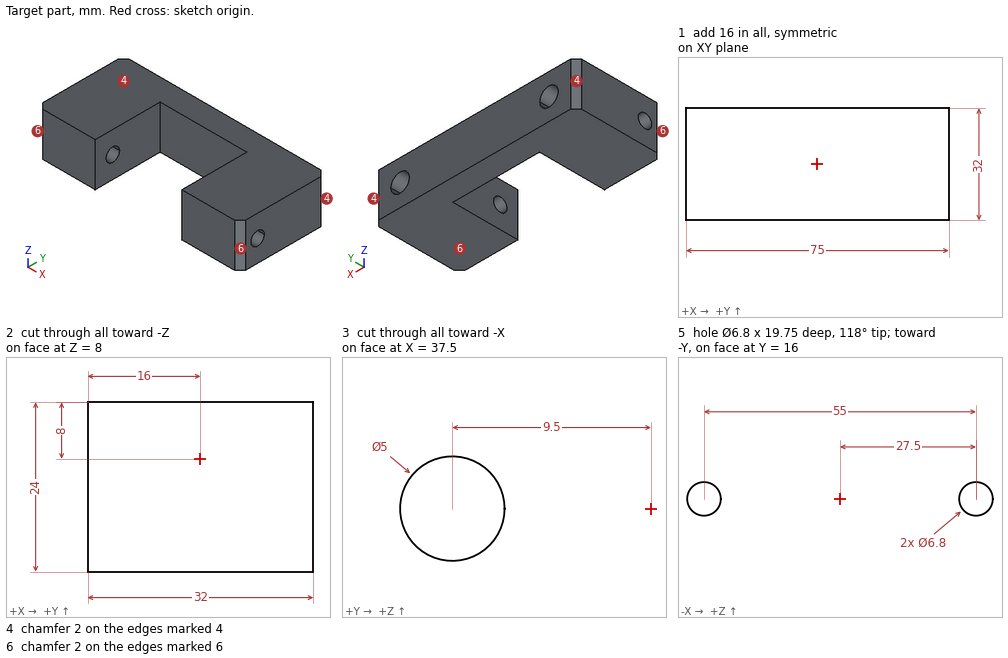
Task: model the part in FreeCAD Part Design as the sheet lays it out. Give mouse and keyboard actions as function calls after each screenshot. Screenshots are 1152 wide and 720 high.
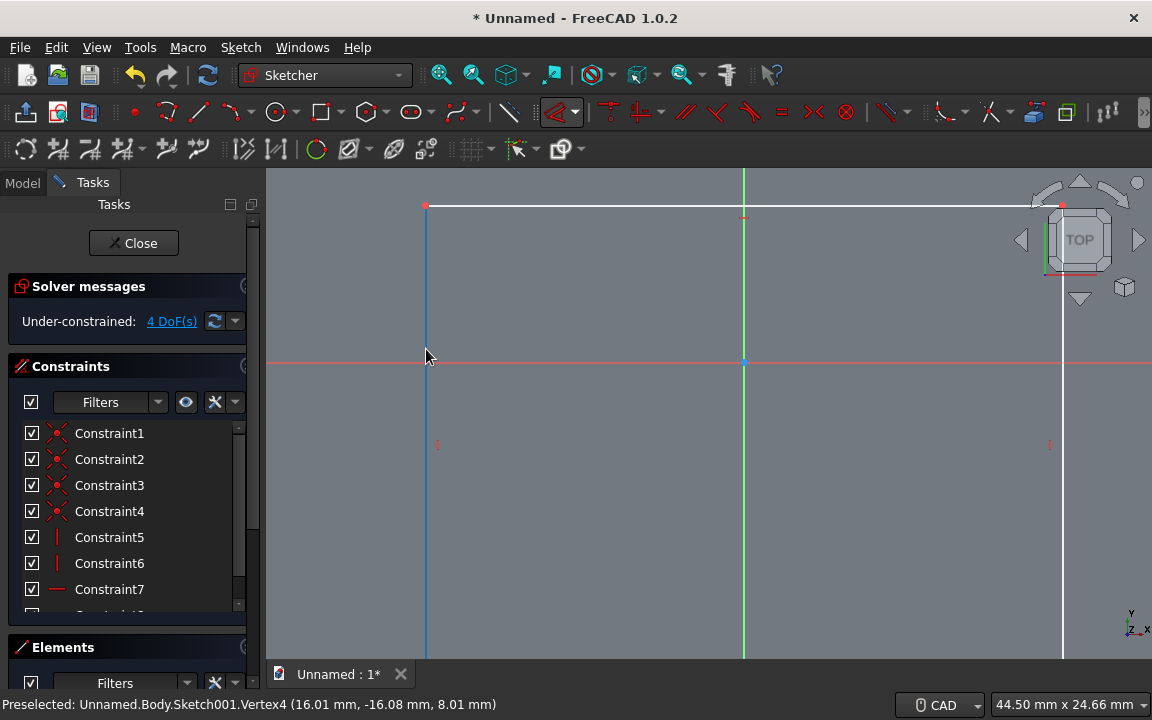
click(426, 349)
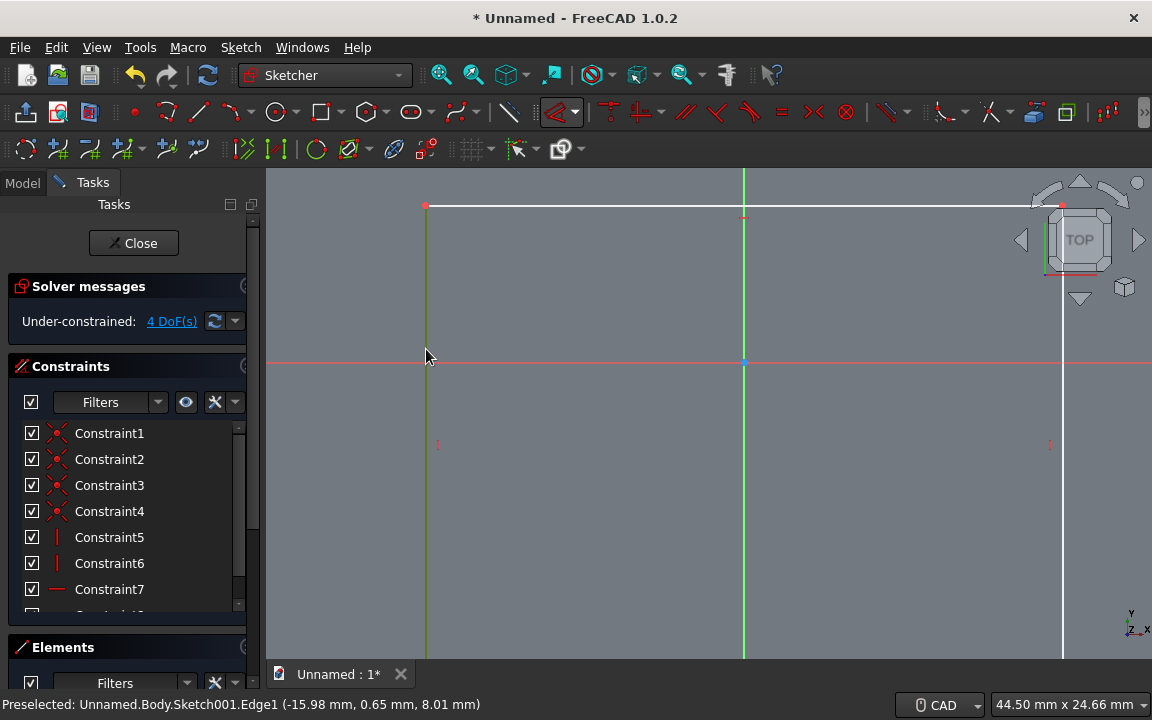
key(i)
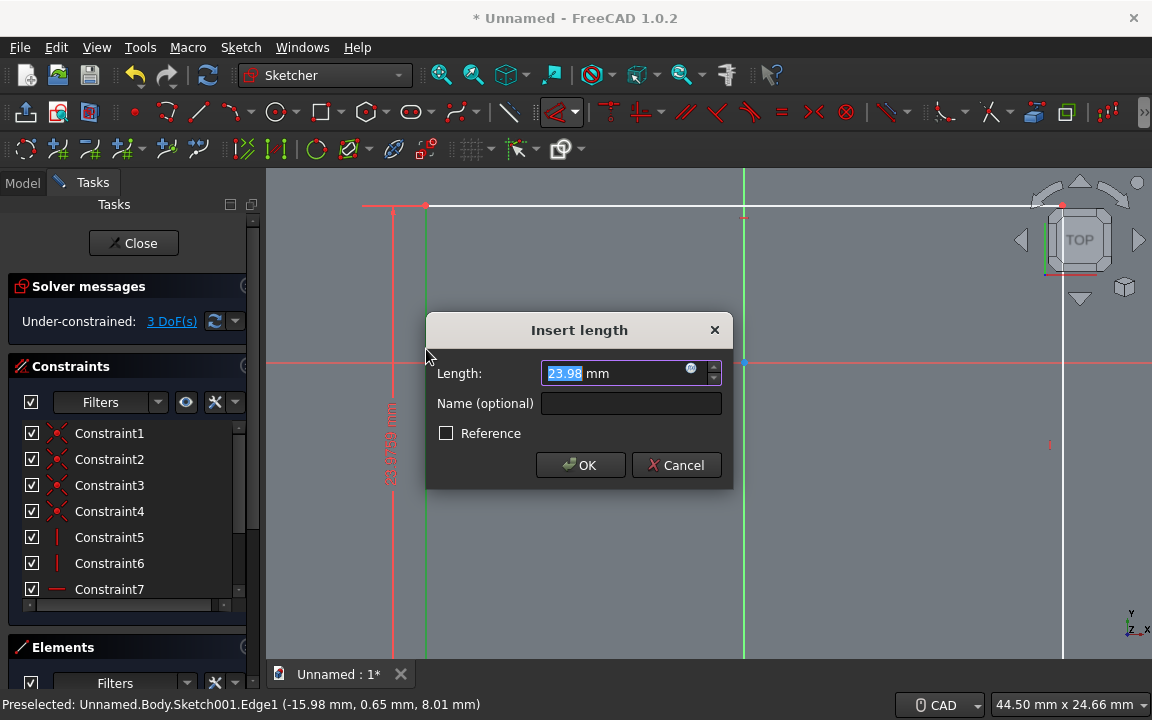
text(24)
key(Return)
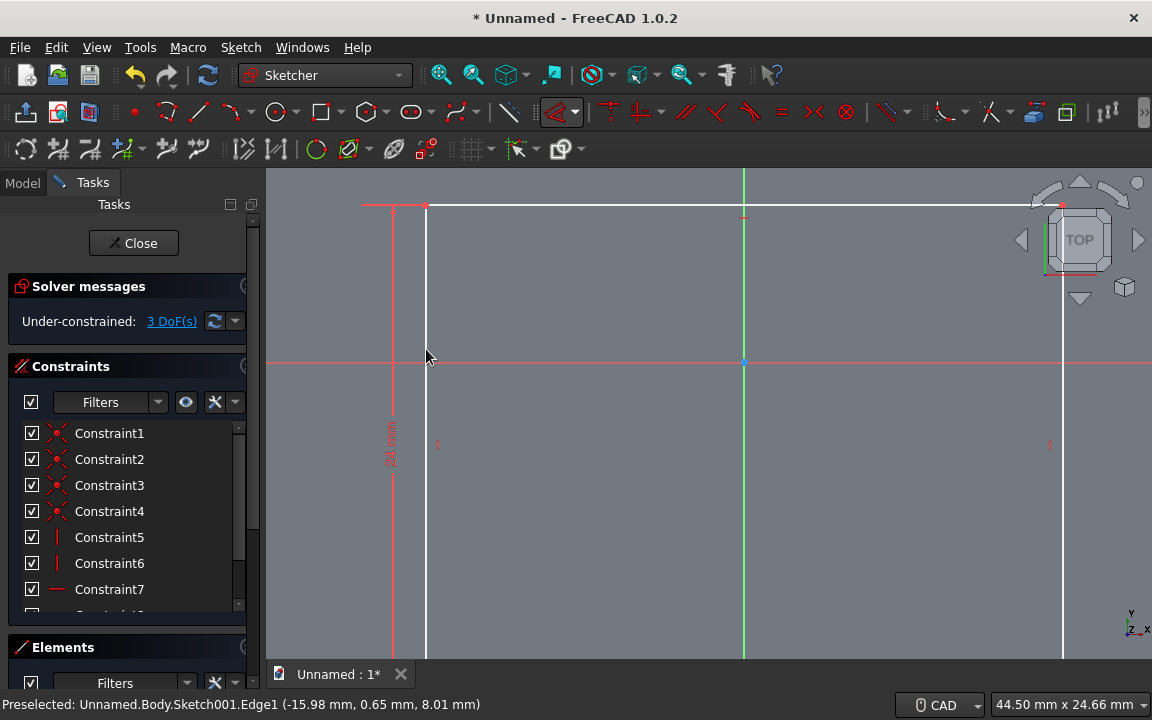
scroll(430, 355, down, 2)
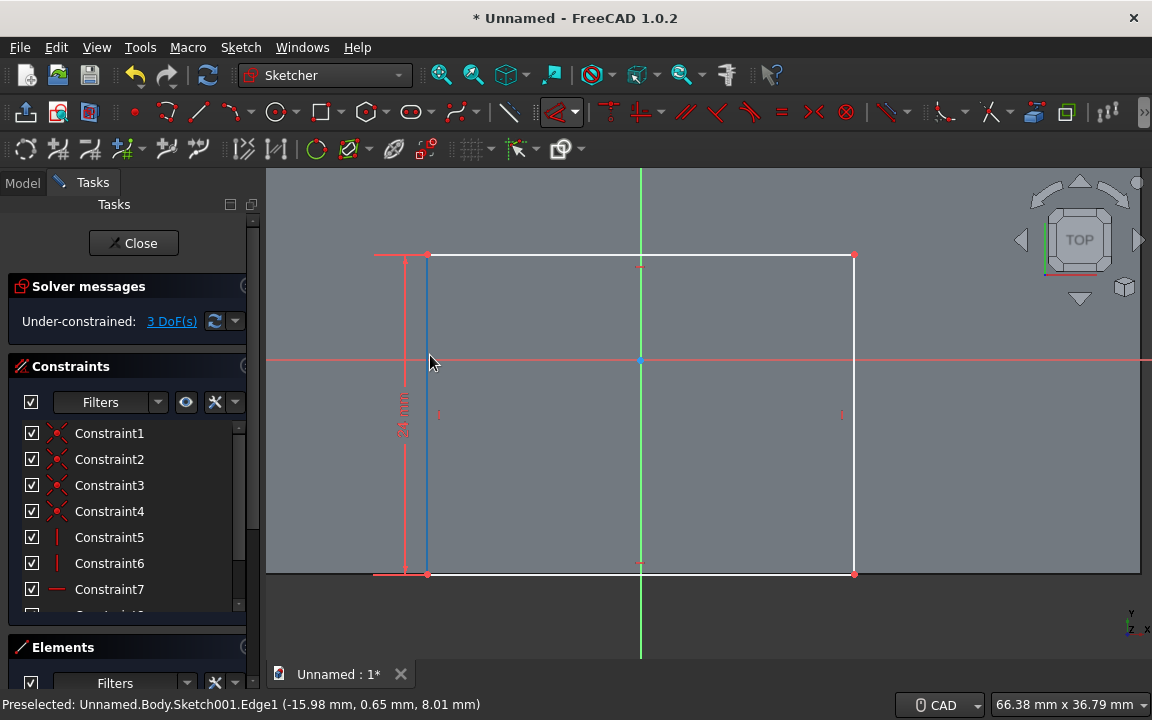
click(555, 575)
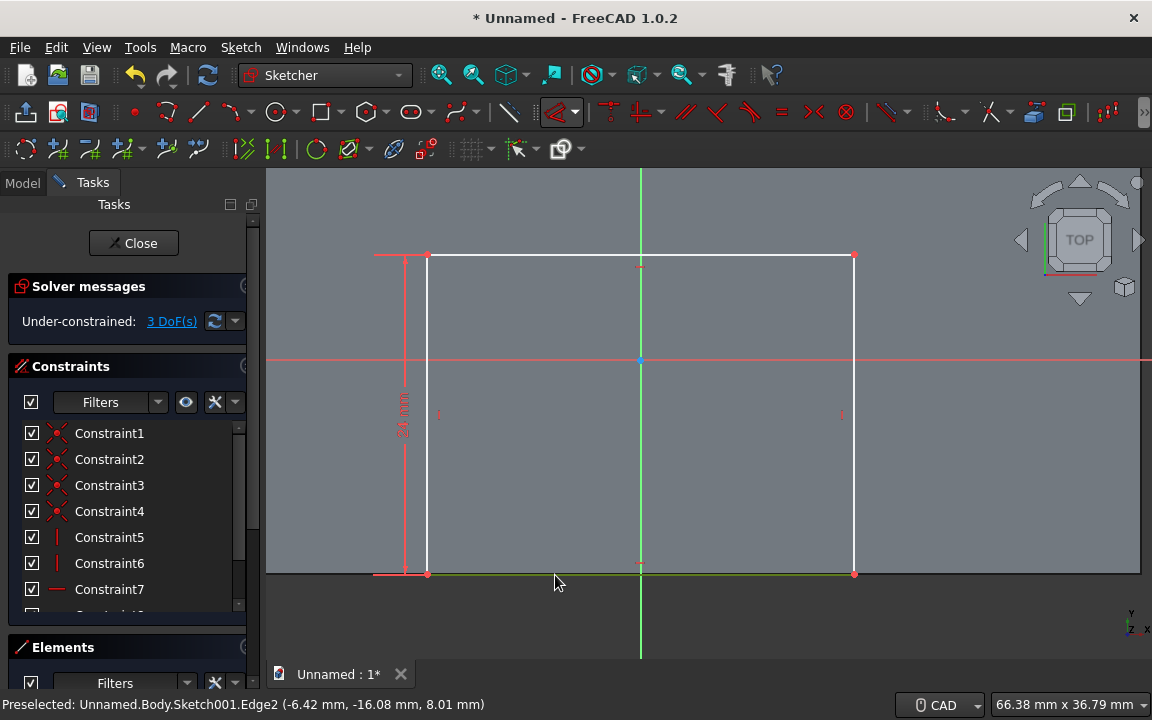
key(l)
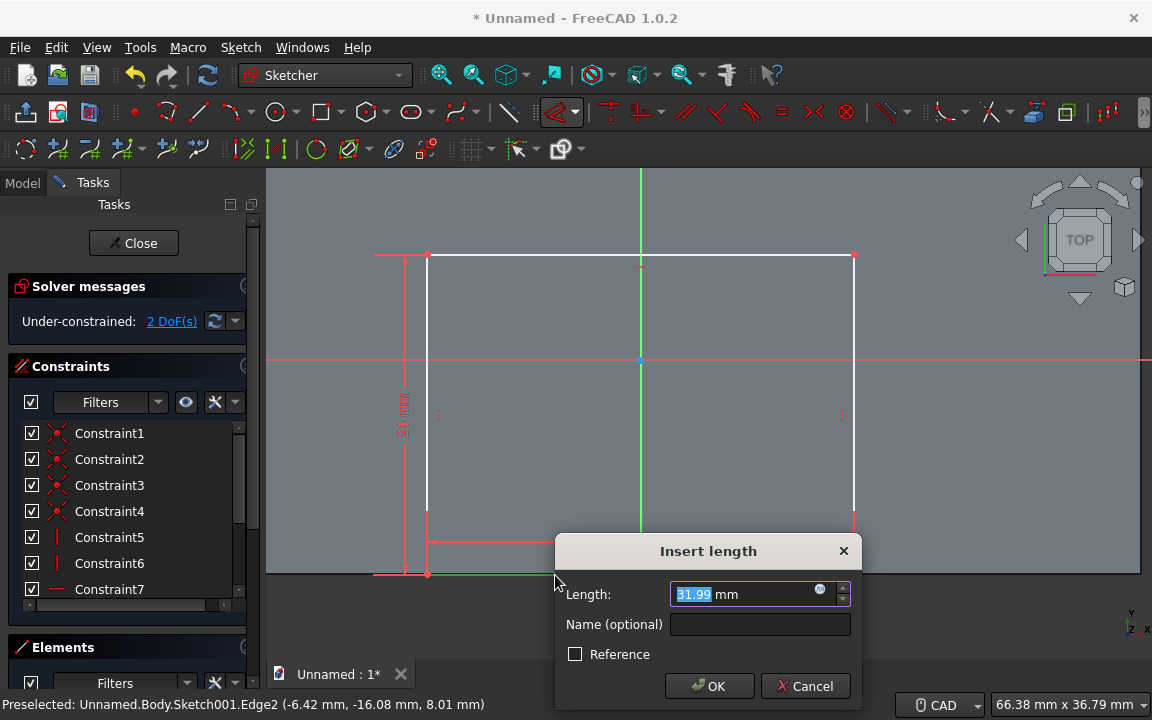
text(32)
key(Return)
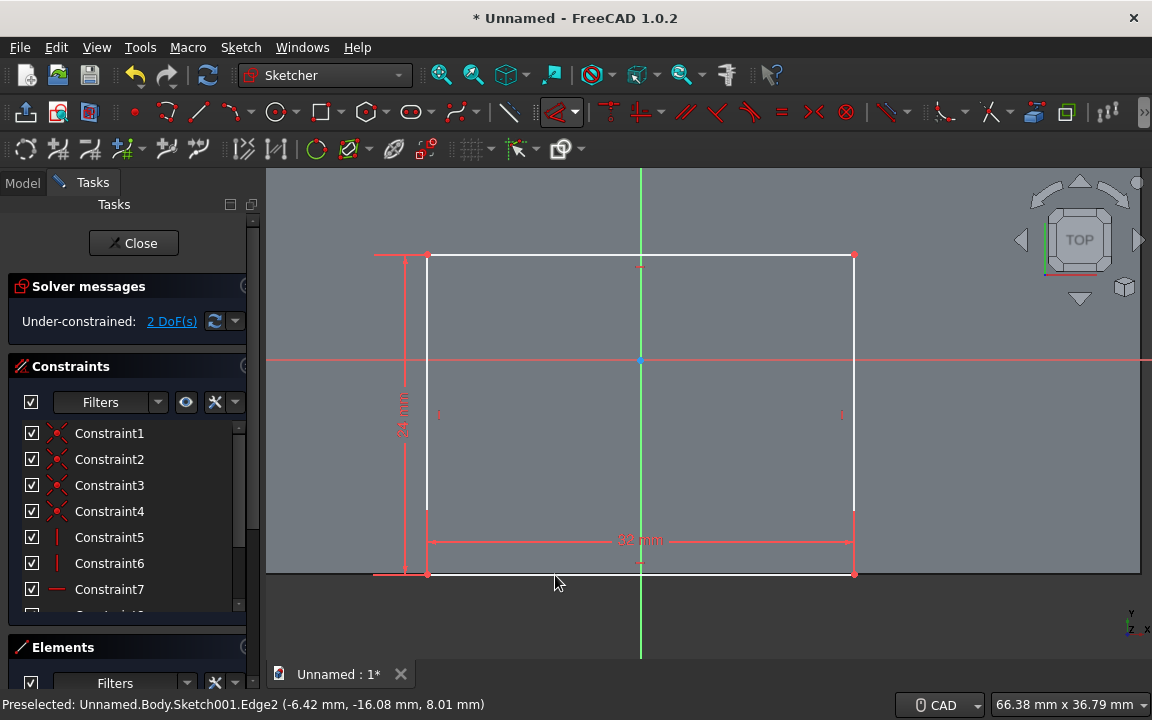
click(427, 255)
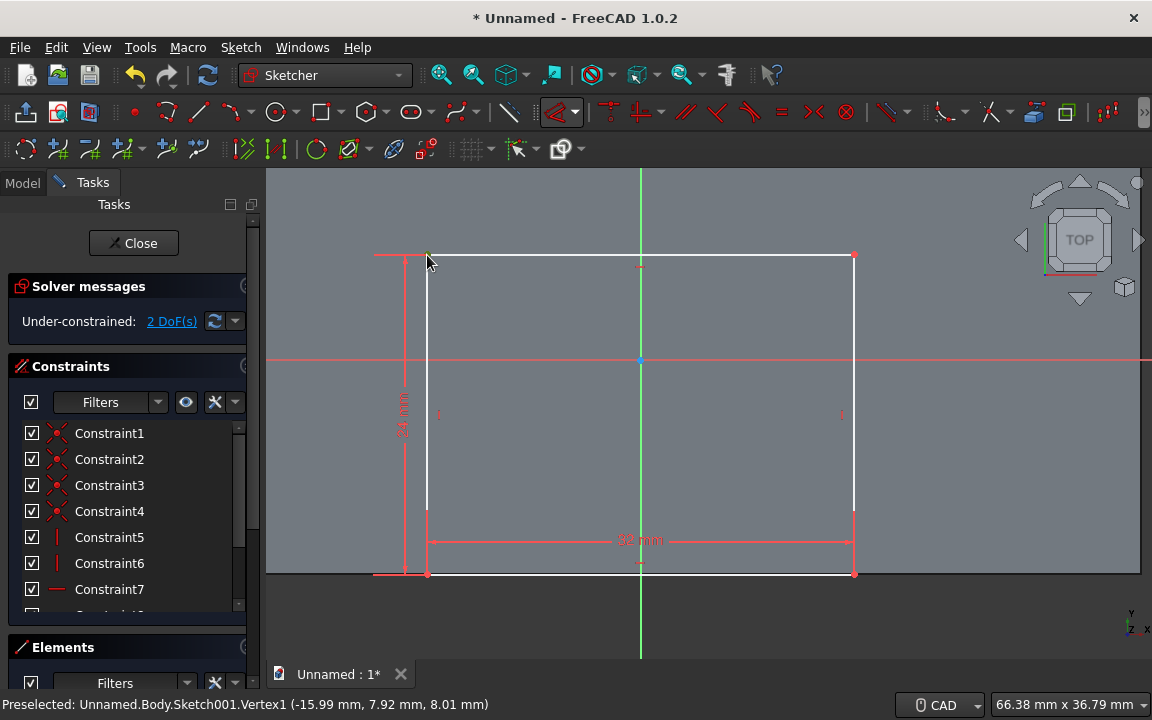
key(i)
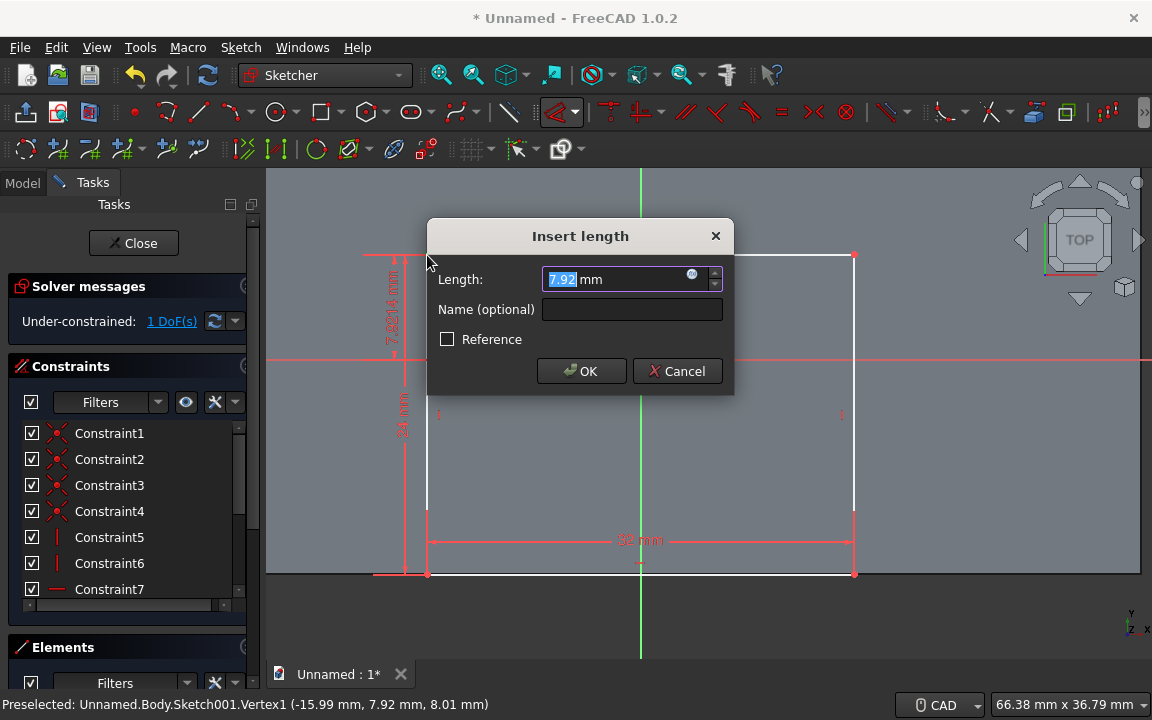
text(8)
key(Return)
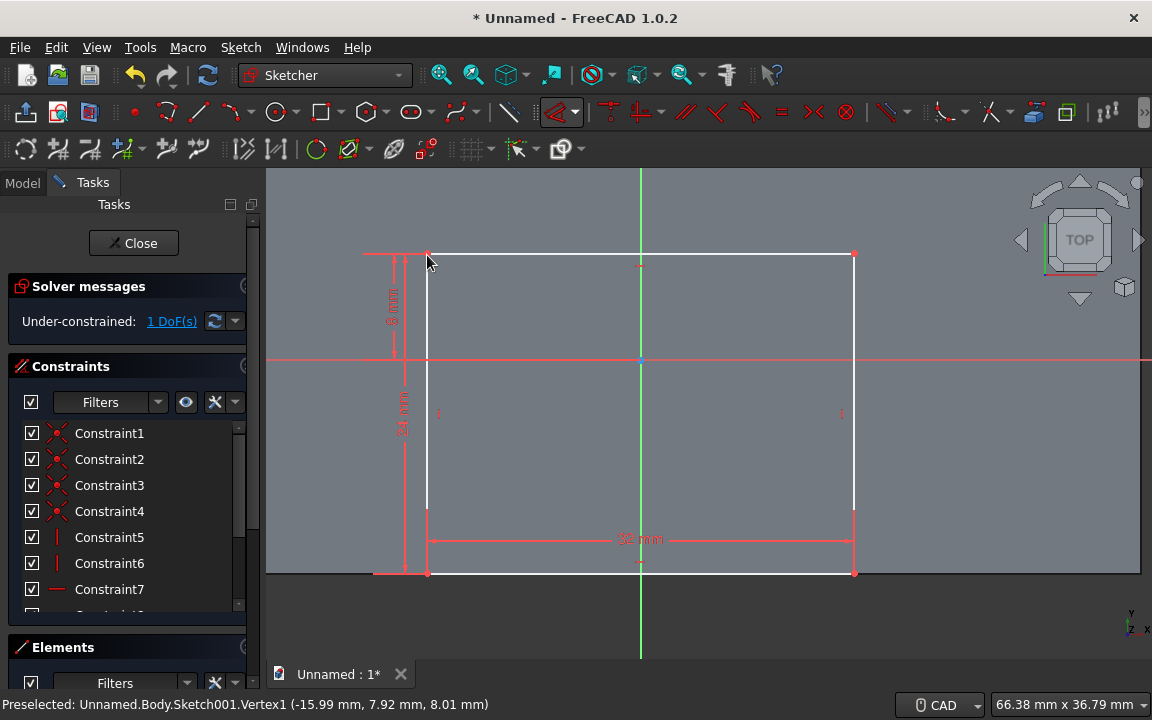
click(427, 254)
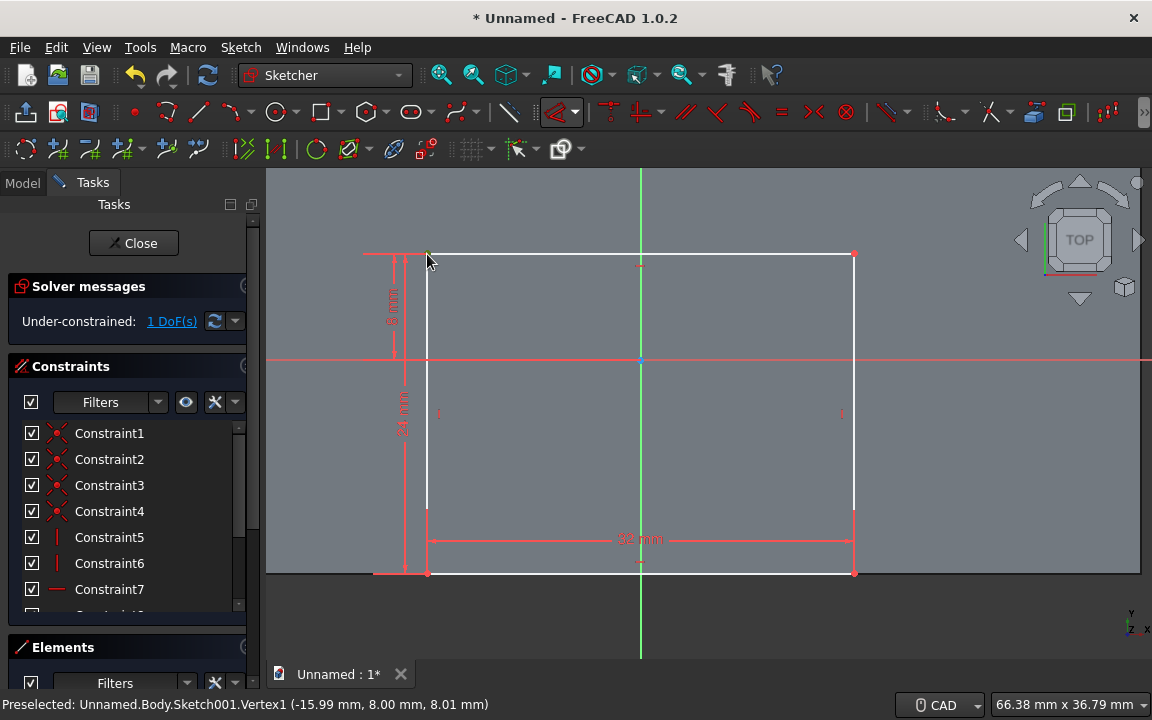
key(l)